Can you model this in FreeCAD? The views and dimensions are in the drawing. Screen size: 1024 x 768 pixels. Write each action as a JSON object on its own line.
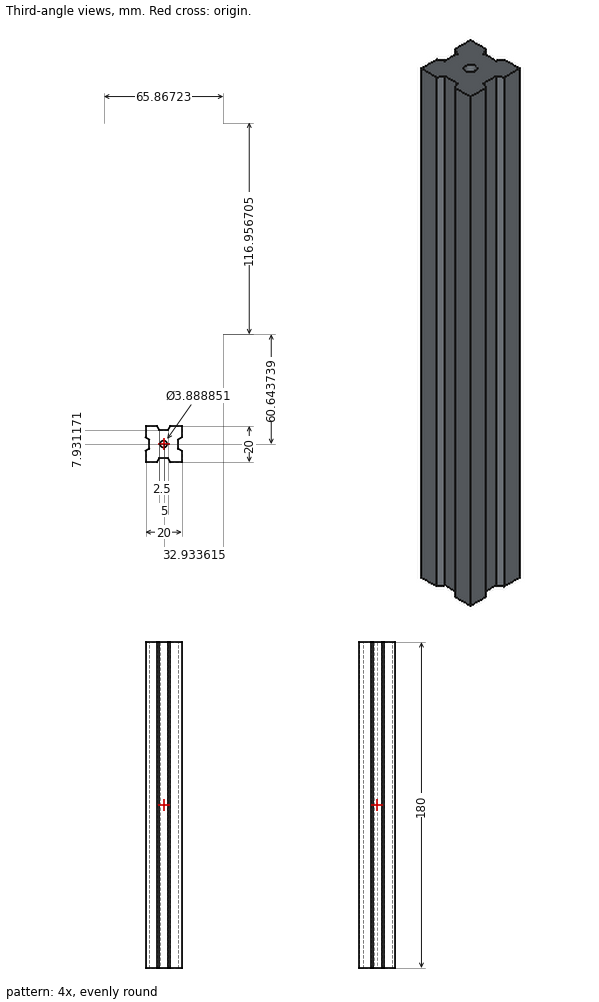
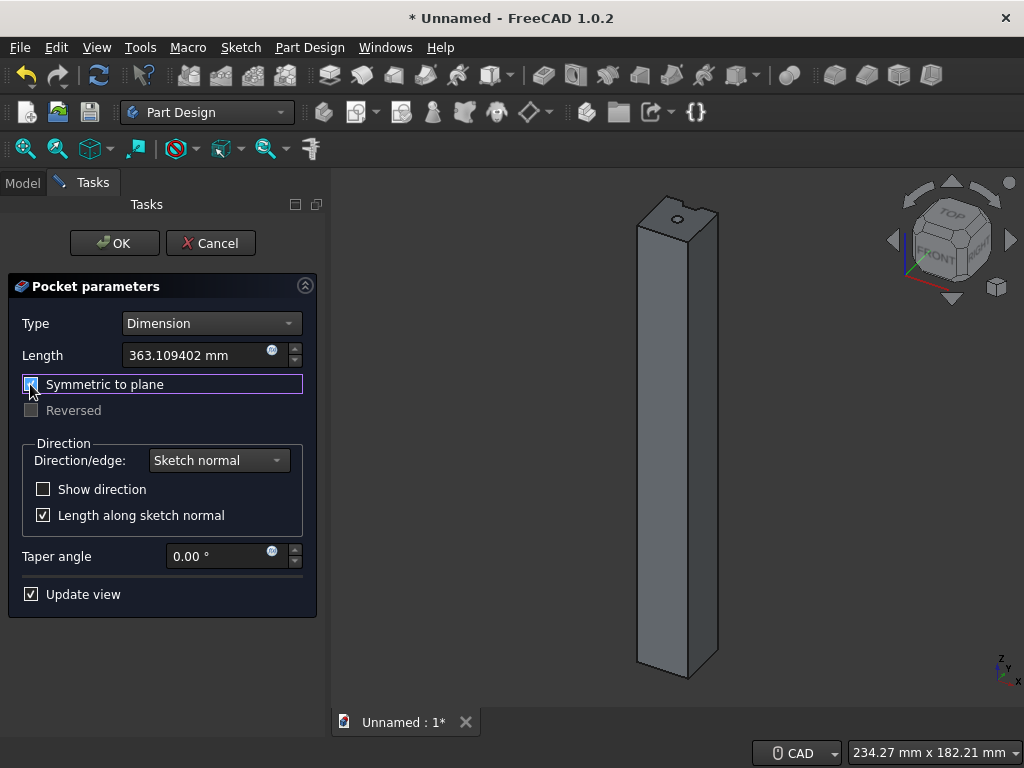
{"action": "left_click", "coordinate": [115, 243]}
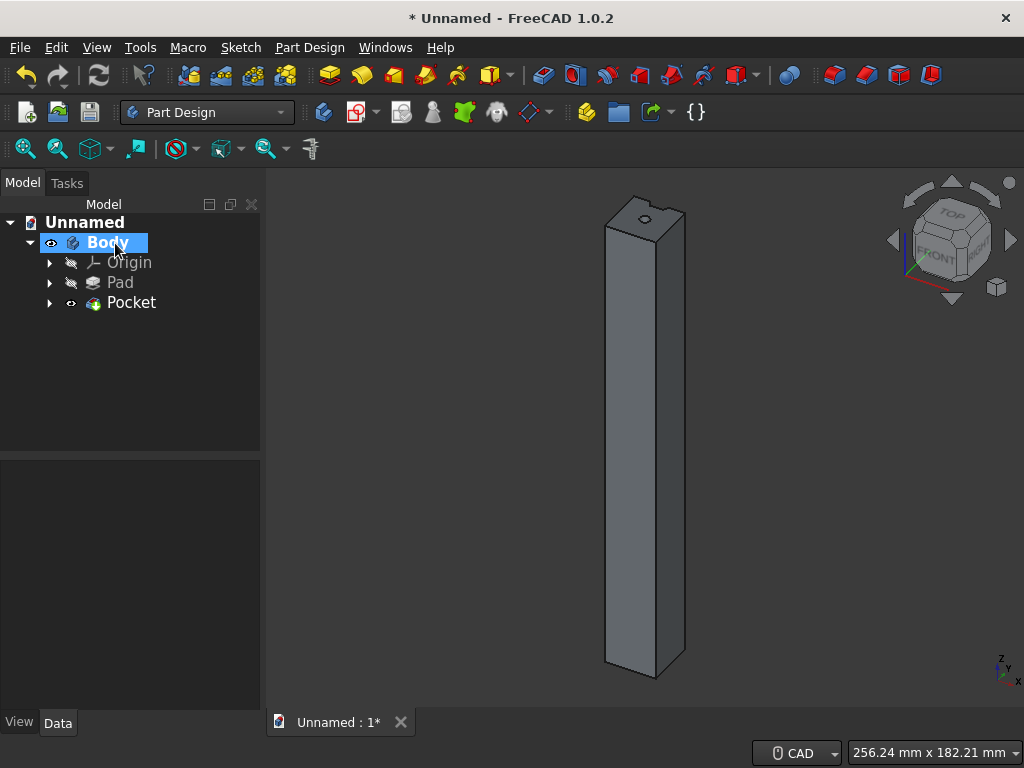
{"action": "left_click", "coordinate": [116, 303]}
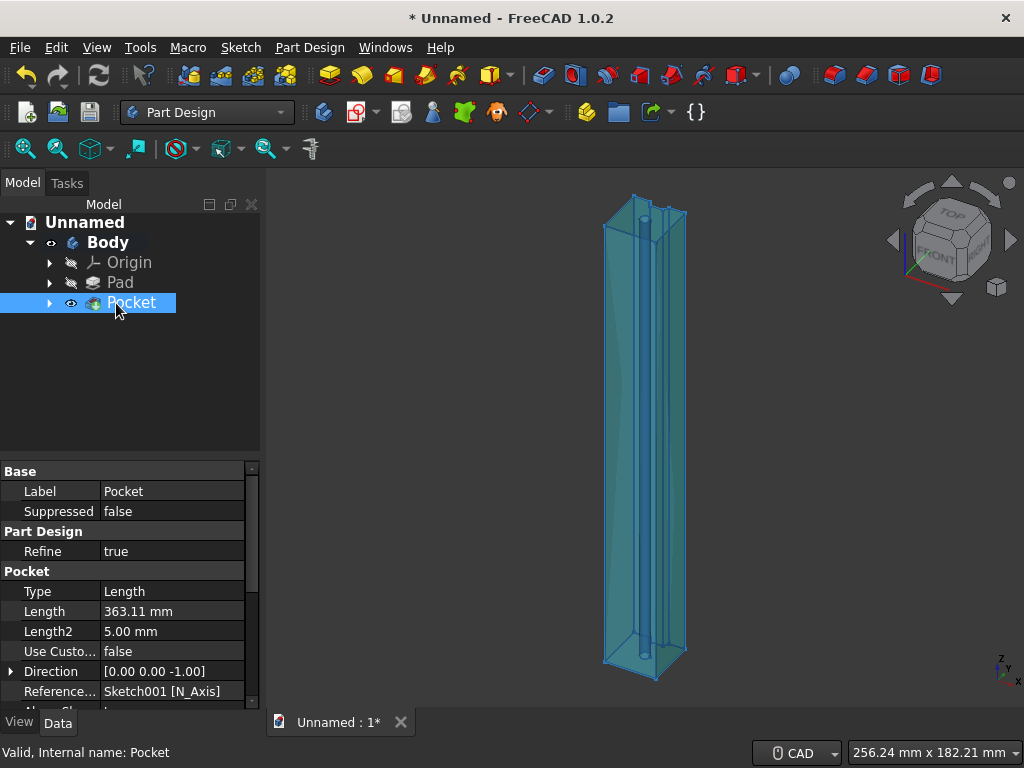
{"action": "left_click", "coordinate": [254, 76]}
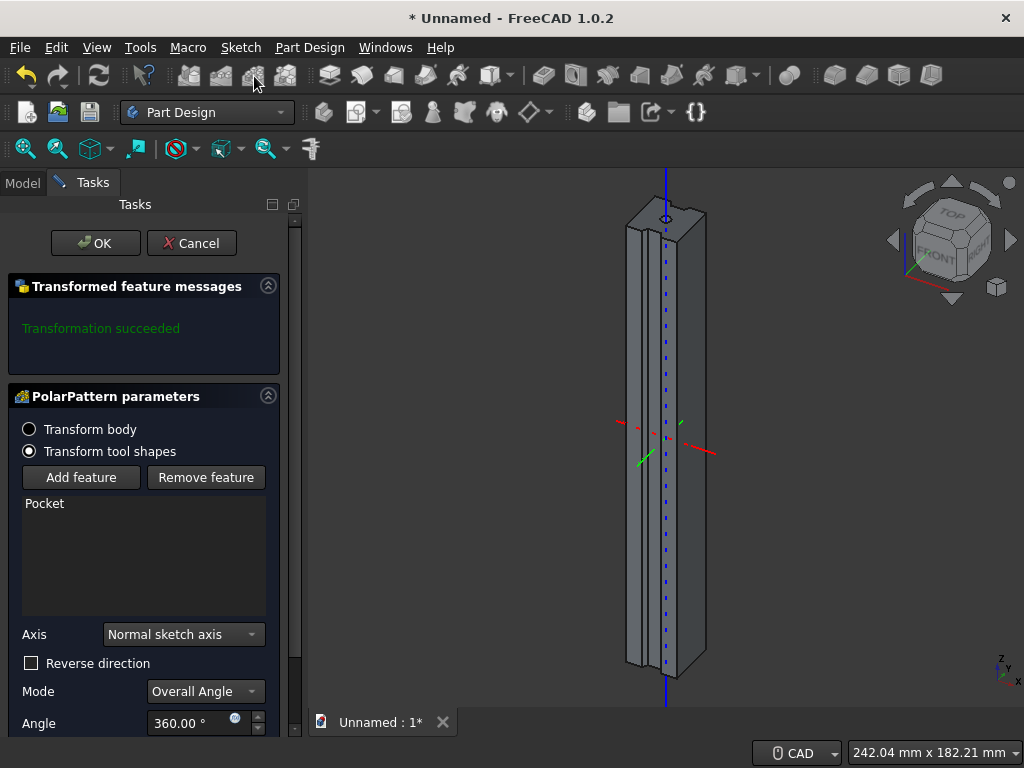
{"action": "left_click", "coordinate": [184, 634]}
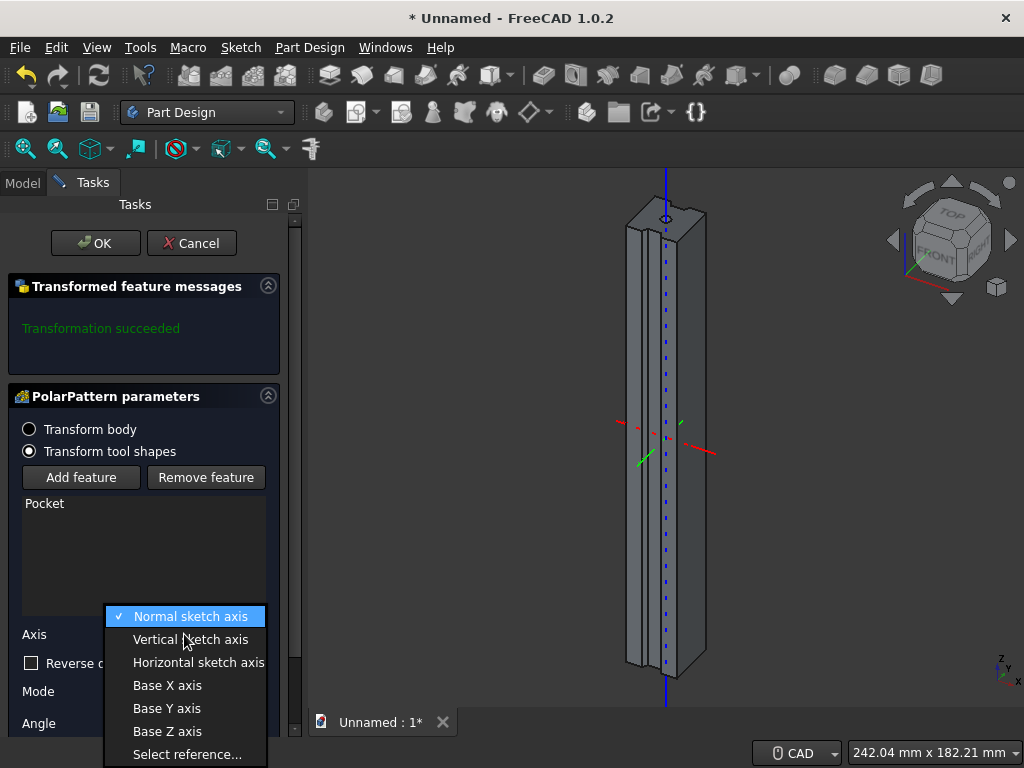
{"action": "left_click", "coordinate": [184, 732]}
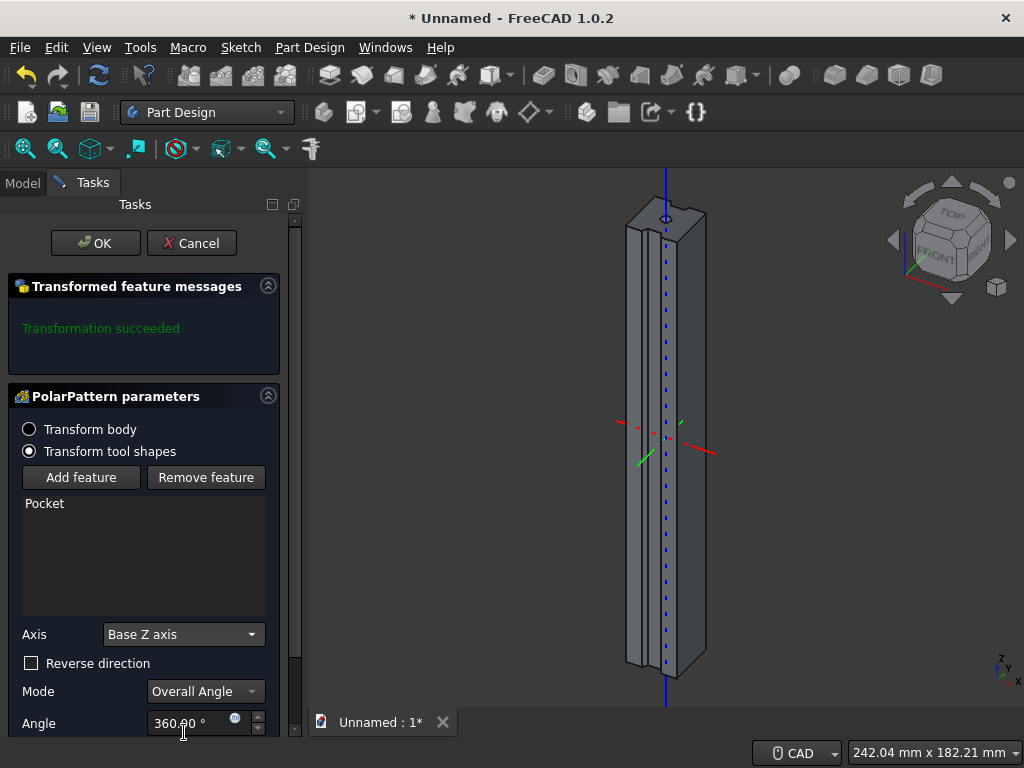
{"action": "scroll", "coordinate": [295, 475], "scroll_direction": "down", "scroll_amount": 2}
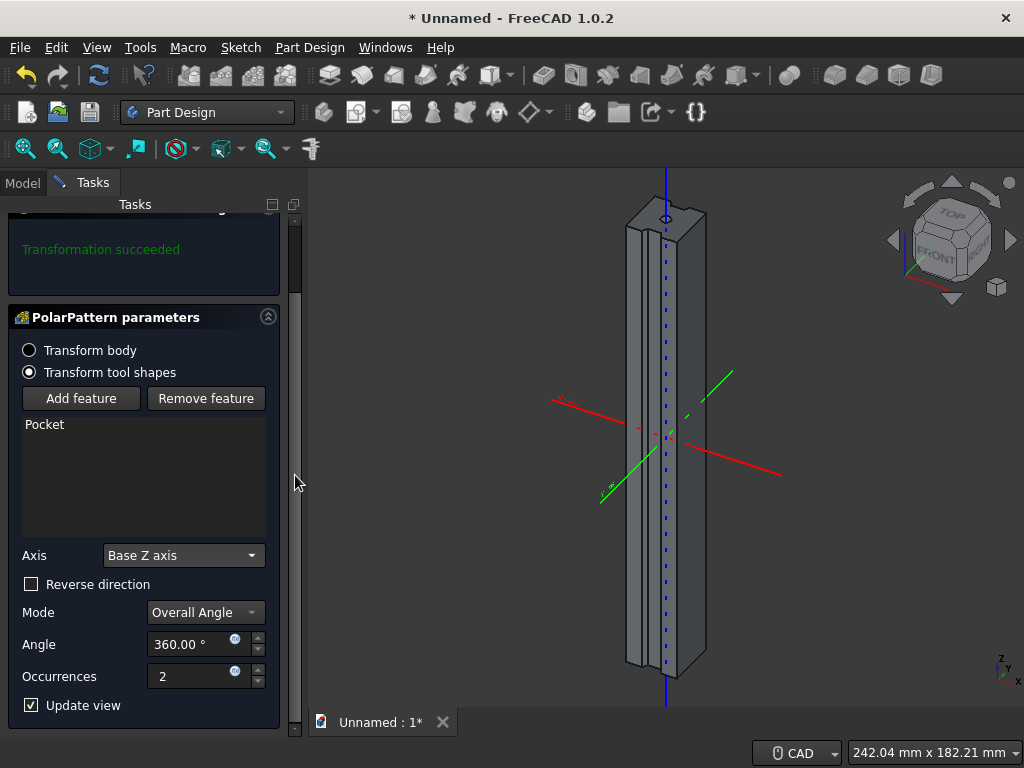
{"action": "triple_click", "coordinate": [198, 676]}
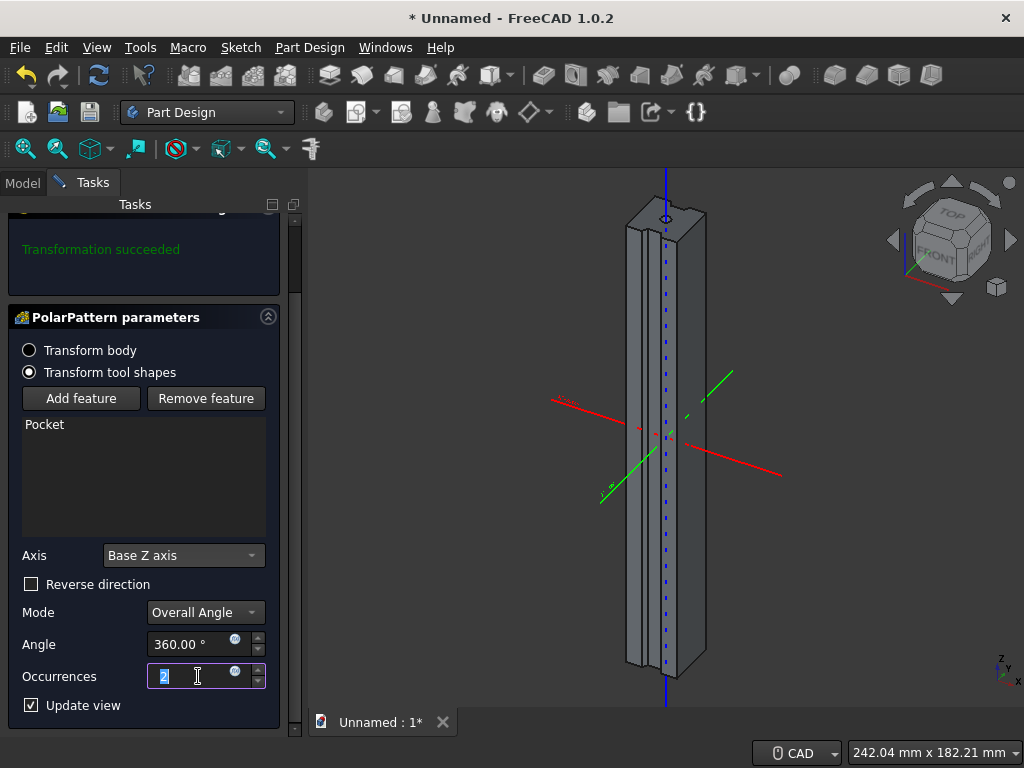
{"action": "type", "text": "4"}
{"action": "key", "text": "Tab"}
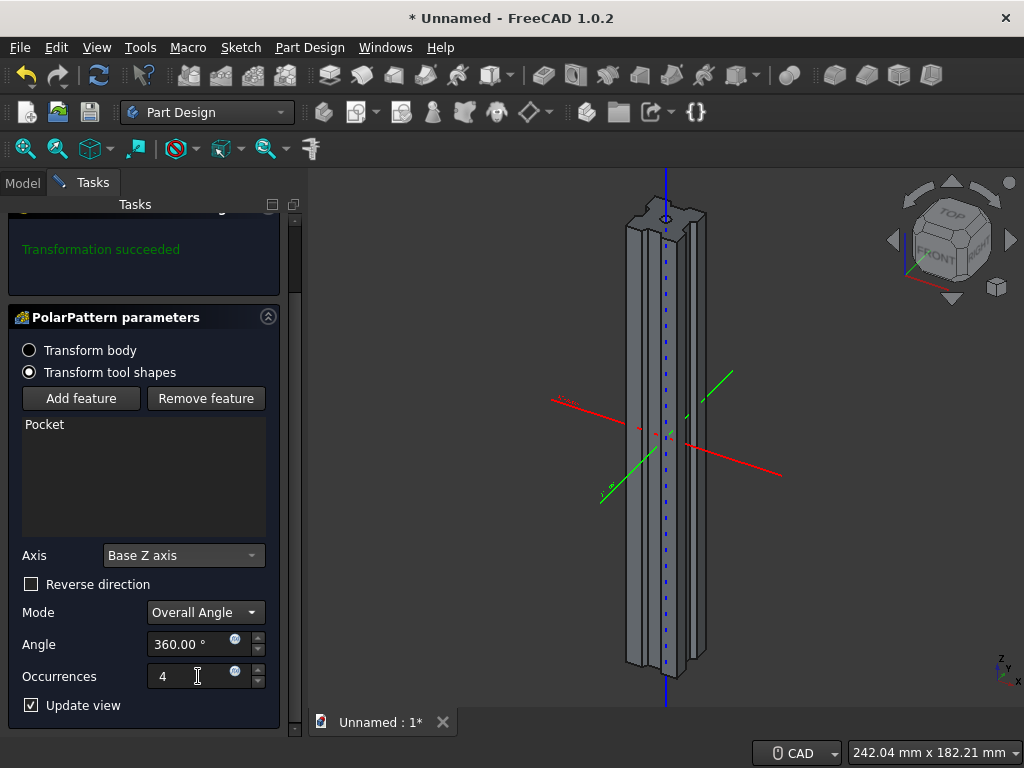
{"action": "scroll", "coordinate": [295, 475], "scroll_direction": "up", "scroll_amount": 3}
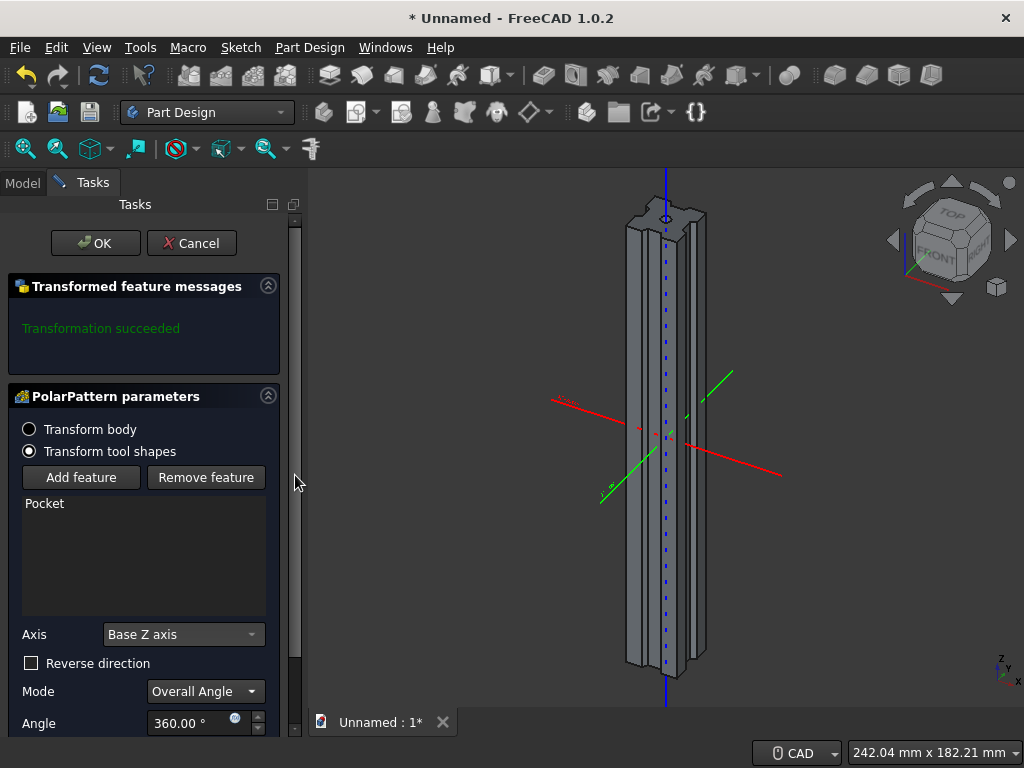
{"action": "left_click", "coordinate": [96, 243]}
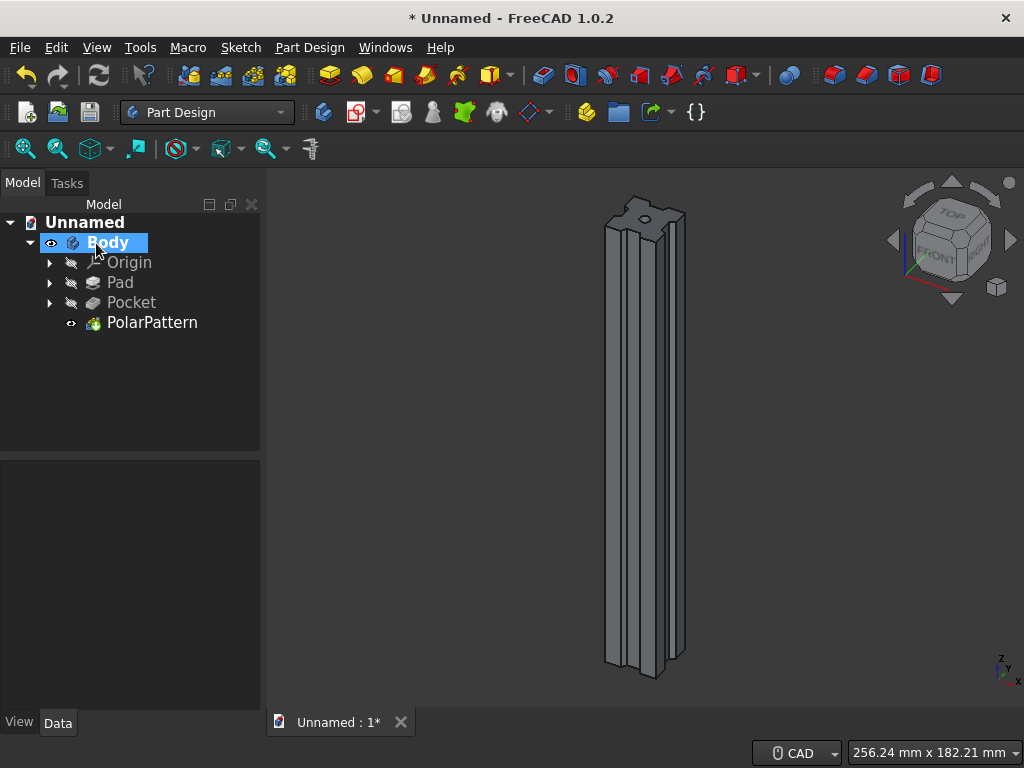
{"action": "key", "text": "0"}